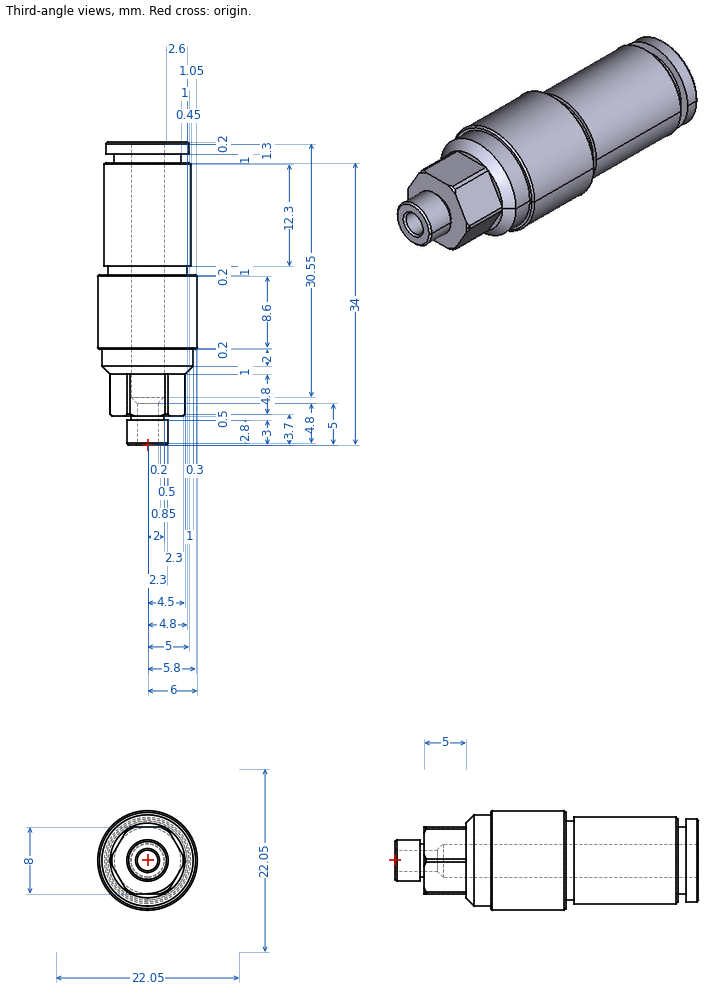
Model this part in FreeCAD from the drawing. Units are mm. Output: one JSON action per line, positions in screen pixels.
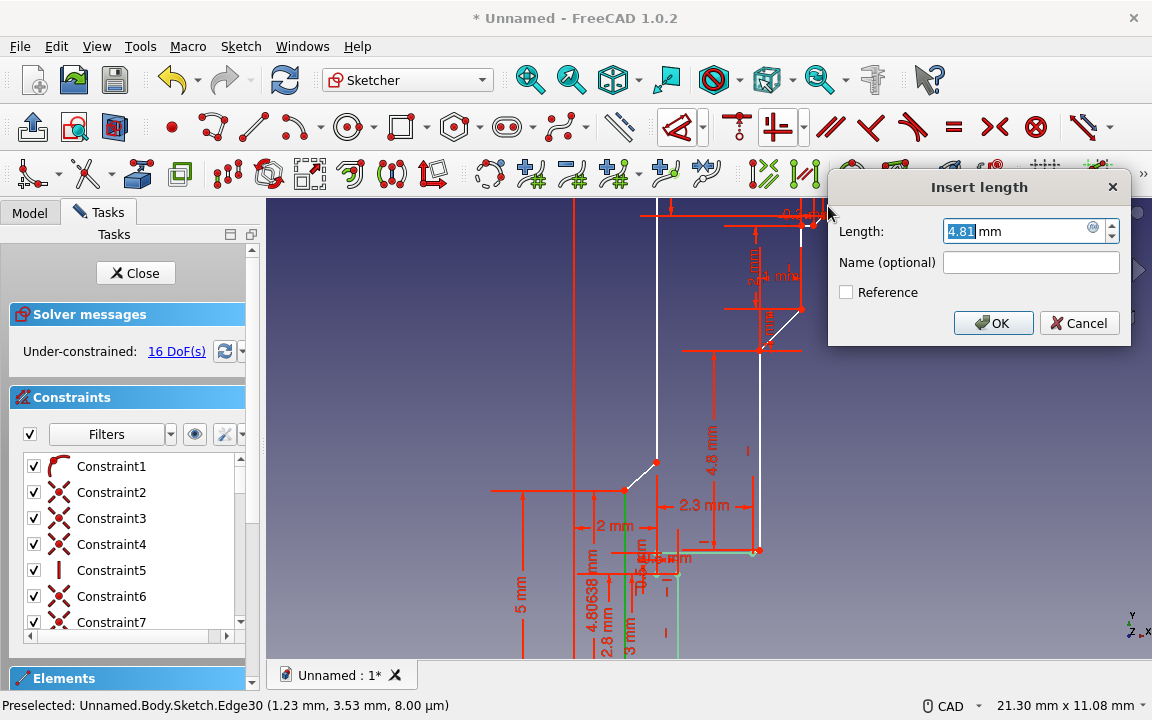
{"action": "type", "text": "4.8"}
{"action": "key", "text": "Return"}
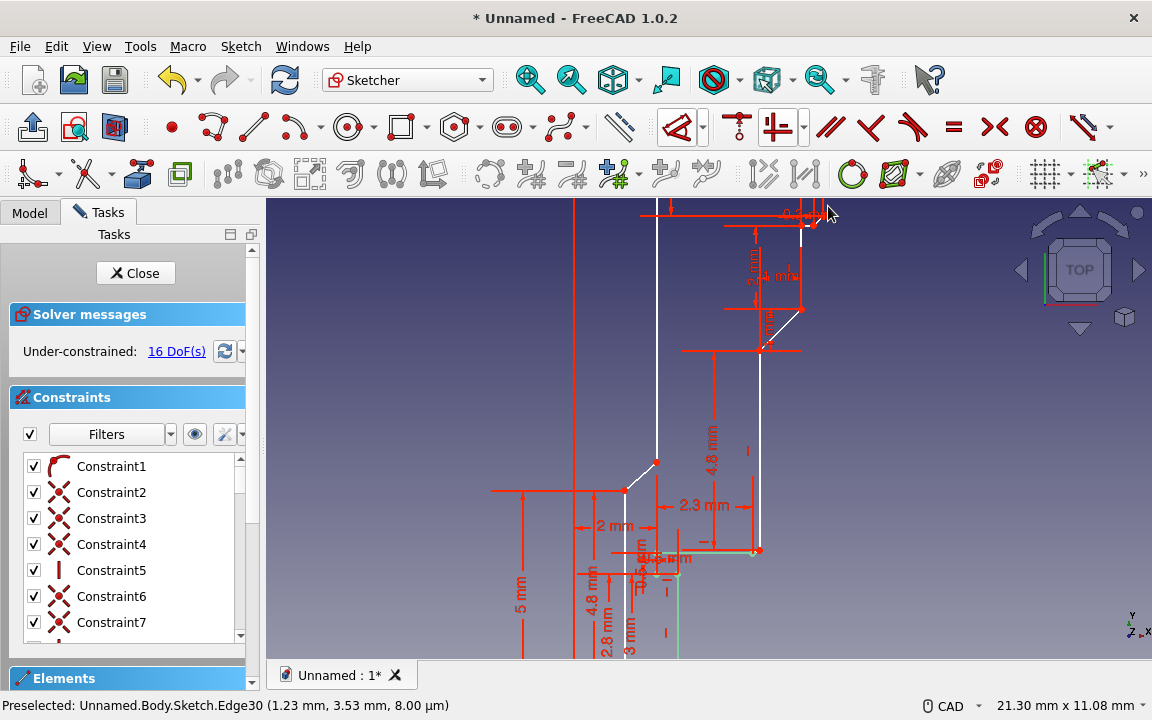
{"action": "scroll", "coordinate": [626, 552], "scroll_direction": "down", "scroll_amount": 8}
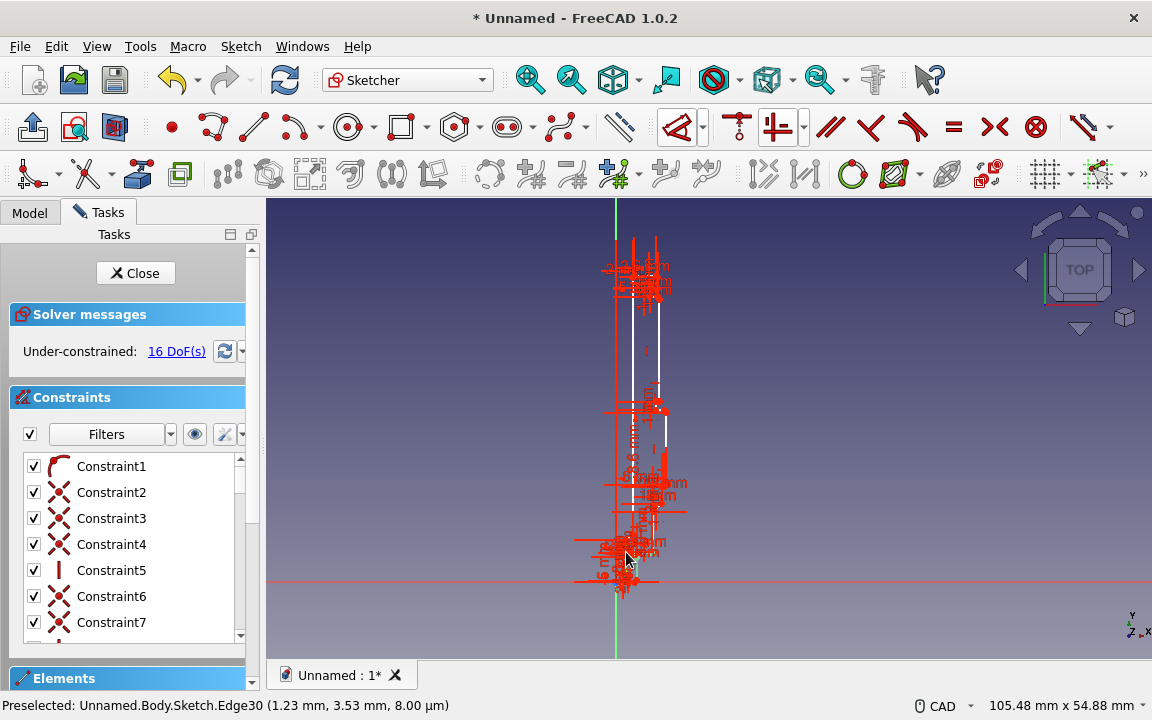
{"action": "scroll", "coordinate": [658, 297], "scroll_direction": "up", "scroll_amount": 7}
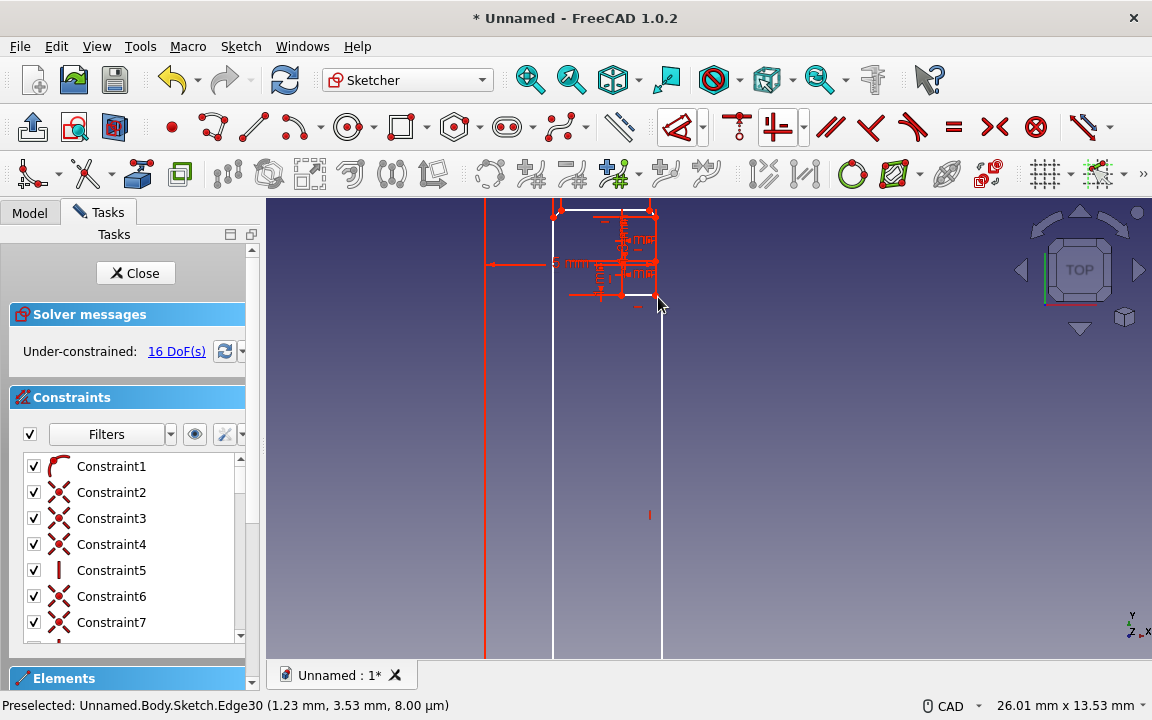
{"action": "left_click", "coordinate": [656, 295]}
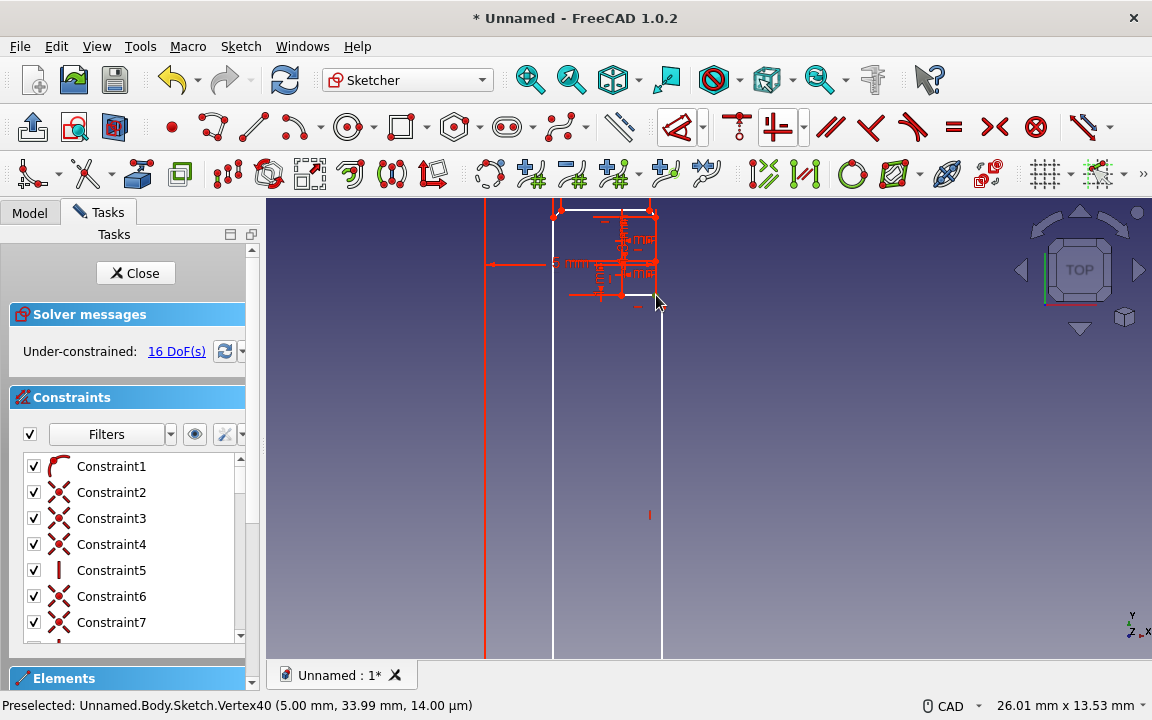
{"action": "left_click", "coordinate": [702, 128]}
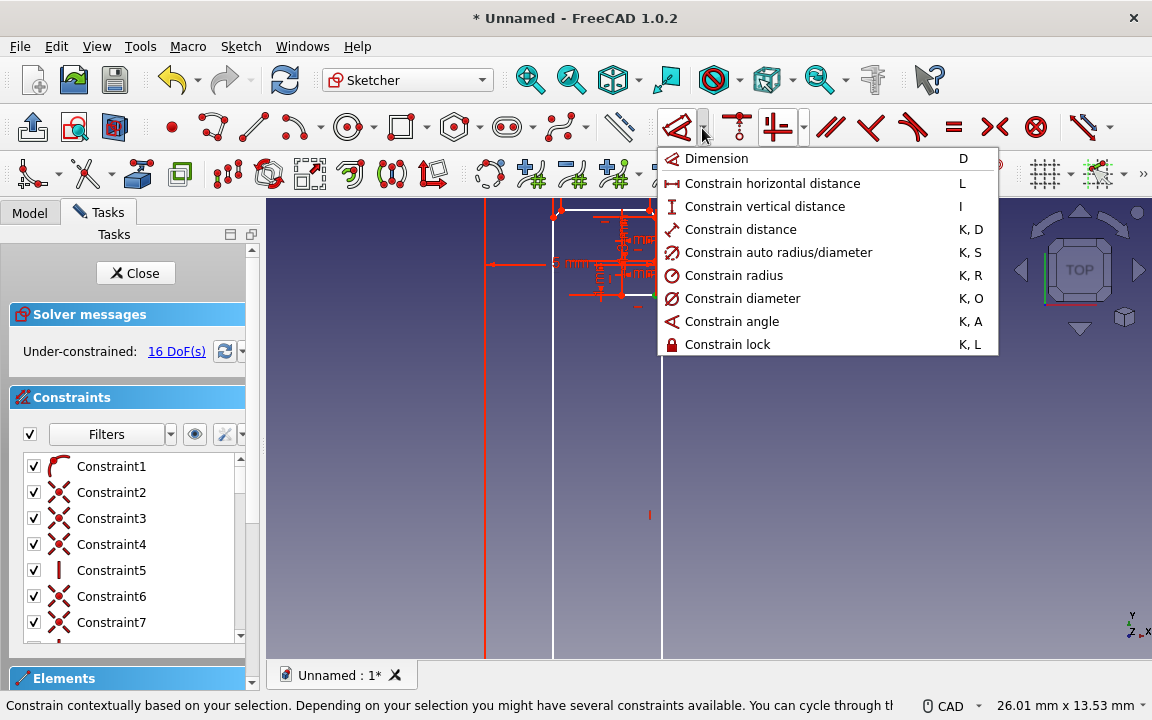
{"action": "left_click", "coordinate": [828, 206]}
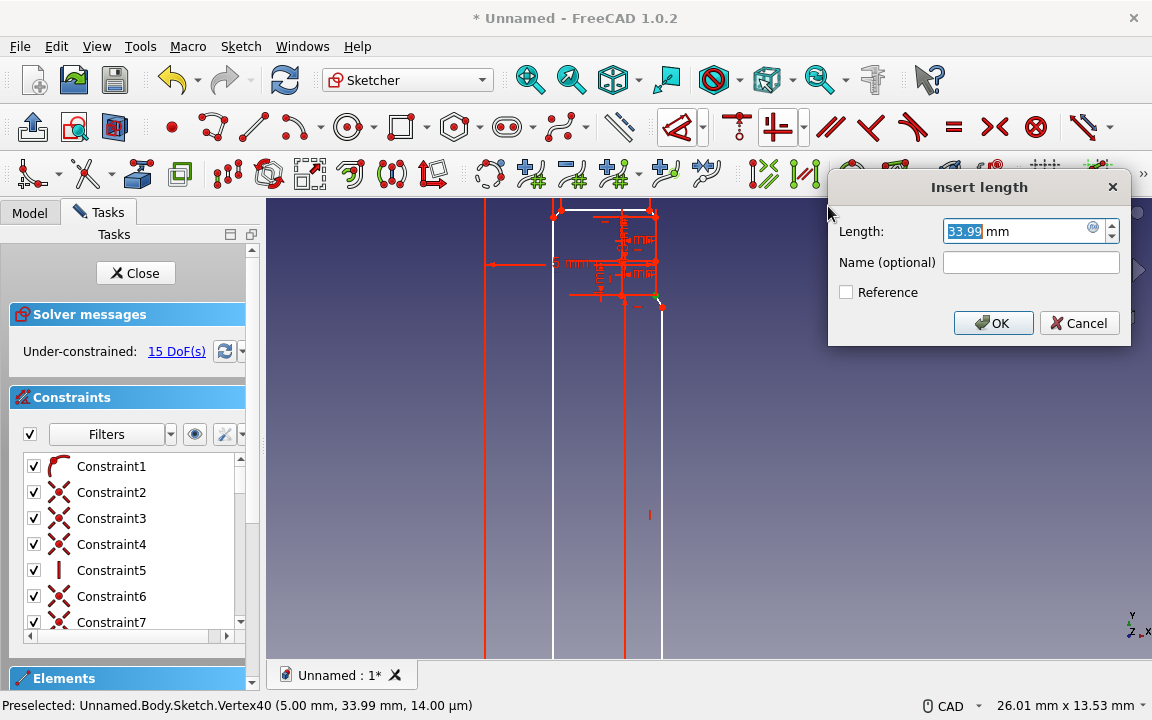
{"action": "type", "text": "34"}
{"action": "key", "text": "Return"}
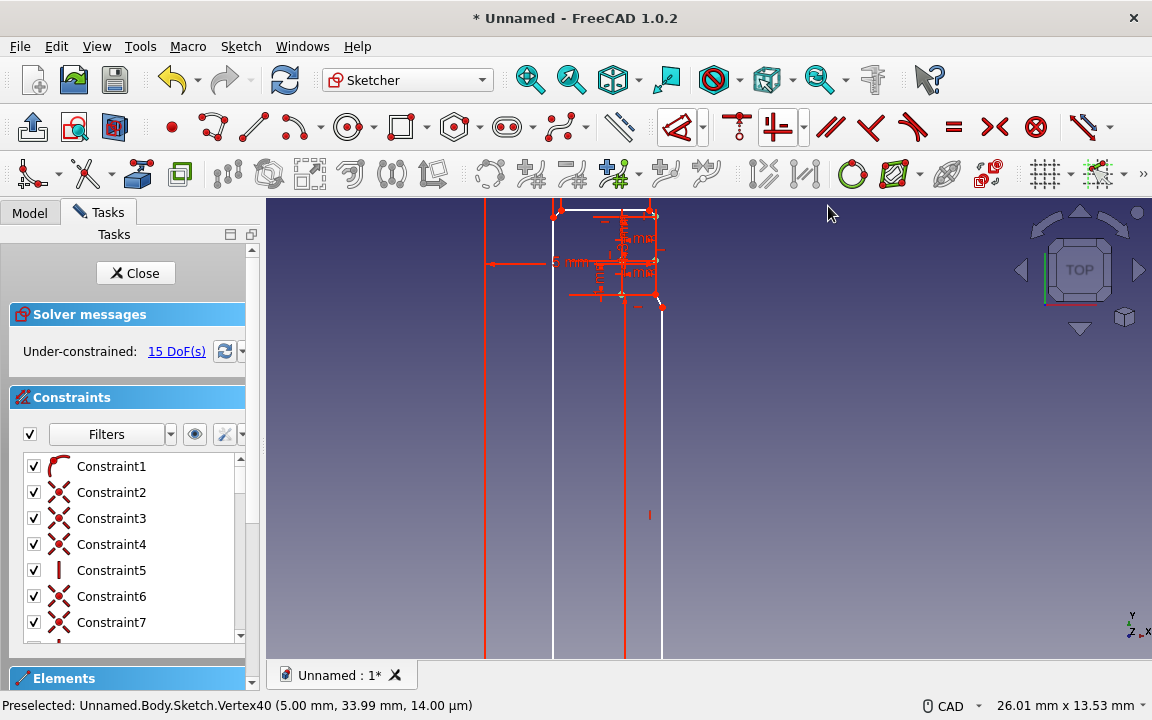
{"action": "scroll", "coordinate": [658, 297], "scroll_direction": "down", "scroll_amount": 7}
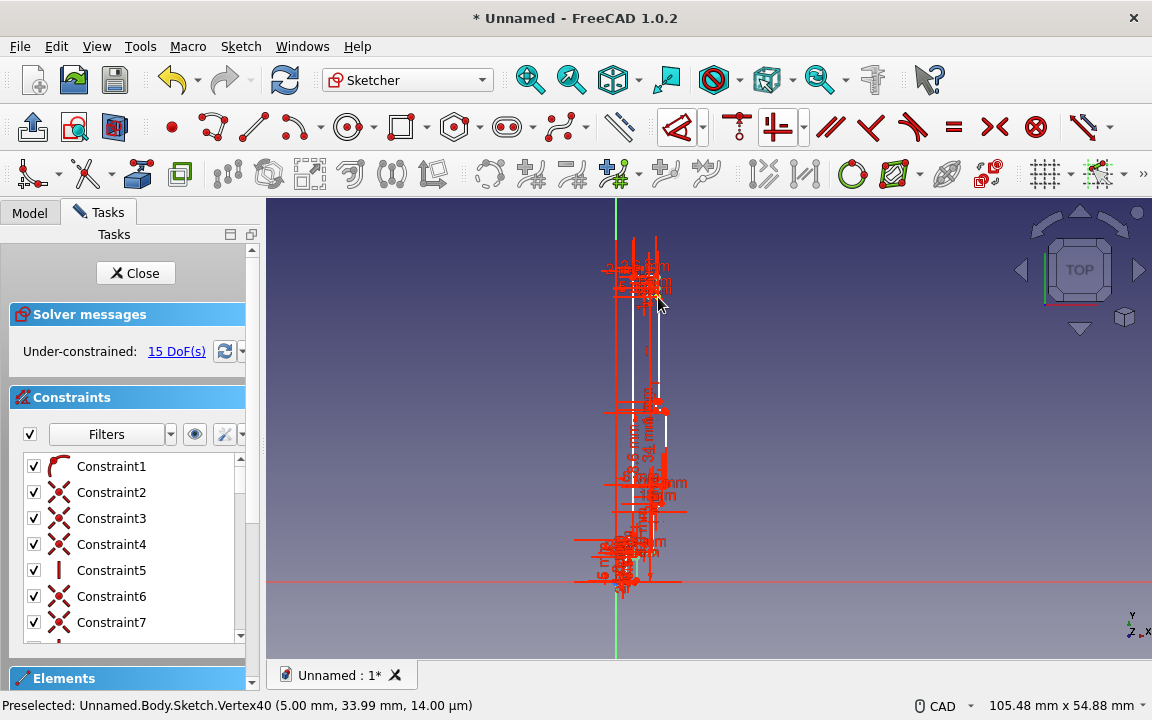
{"action": "scroll", "coordinate": [631, 582], "scroll_direction": "up", "scroll_amount": 9}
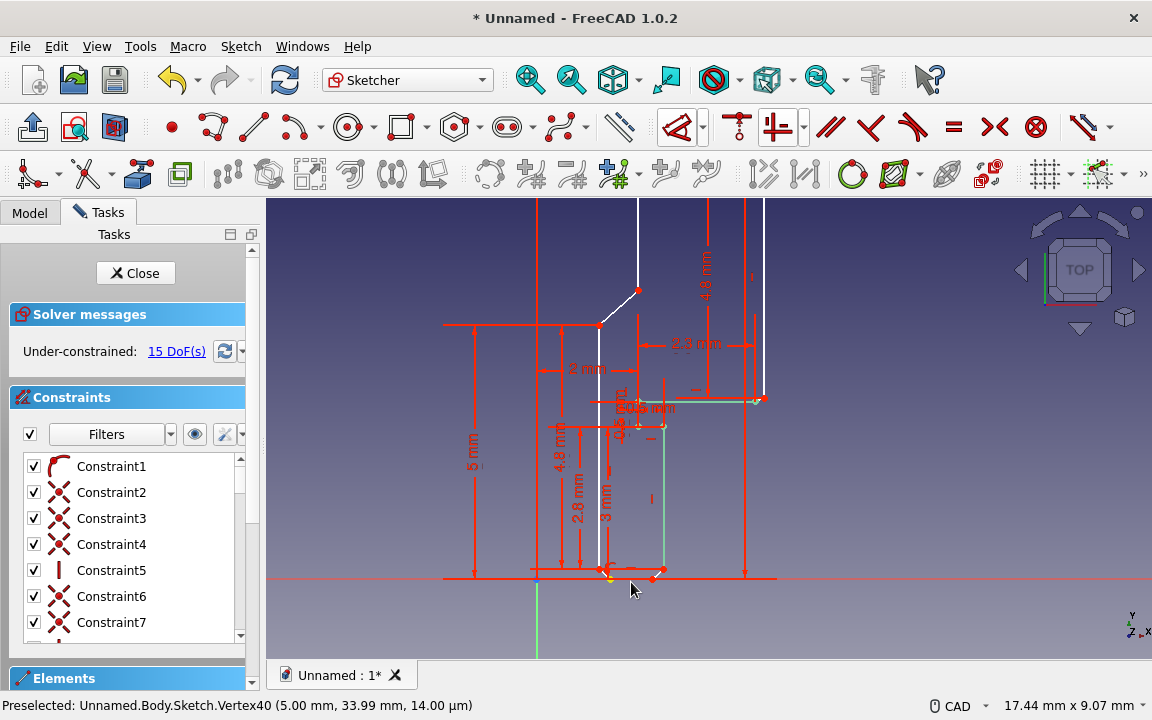
{"action": "left_click", "coordinate": [627, 579]}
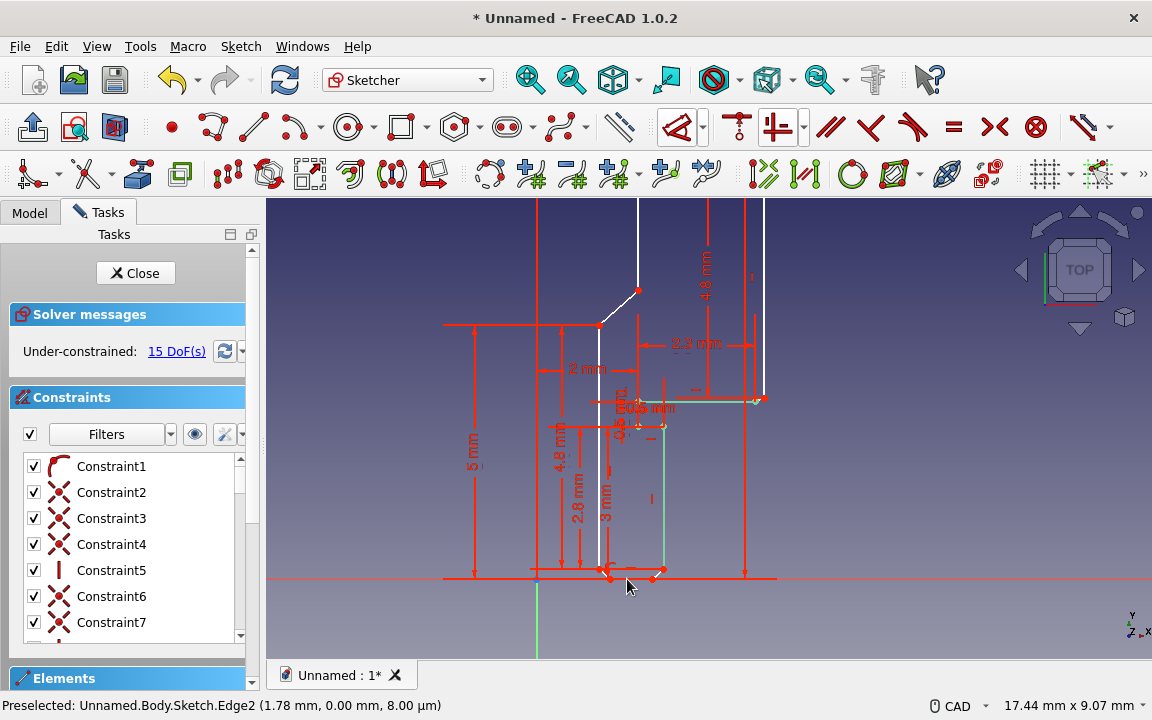
{"action": "key", "text": "l"}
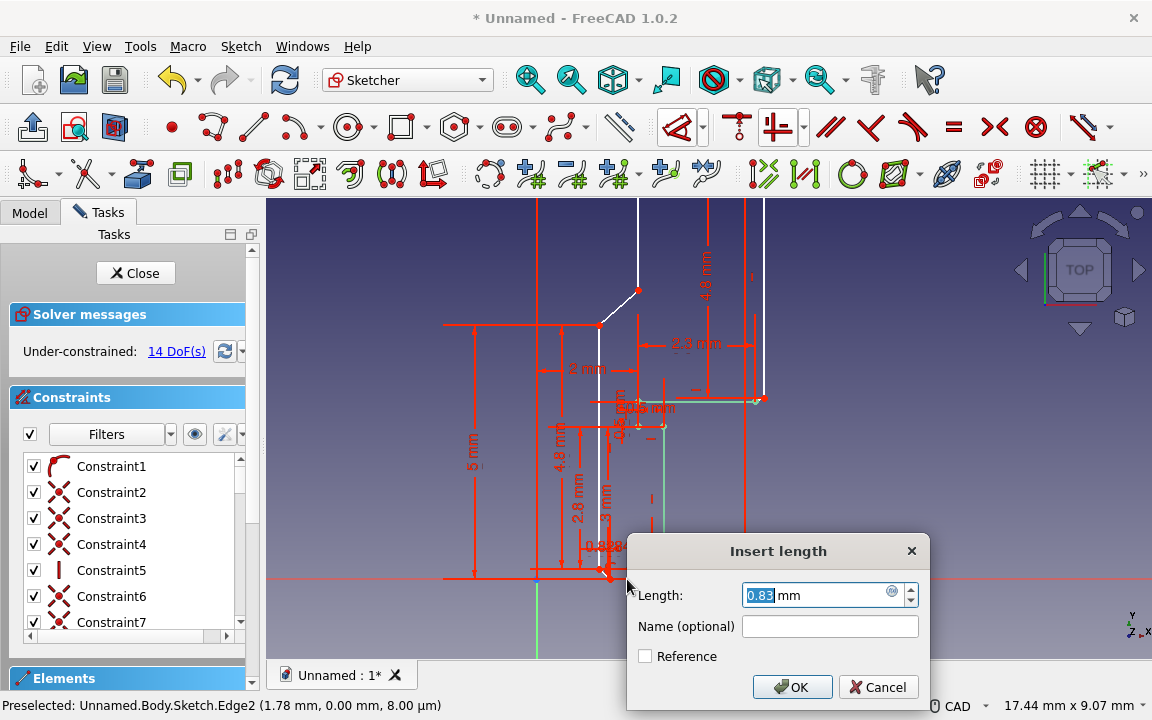
{"action": "type", "text": "0.85"}
{"action": "key", "text": "Return"}